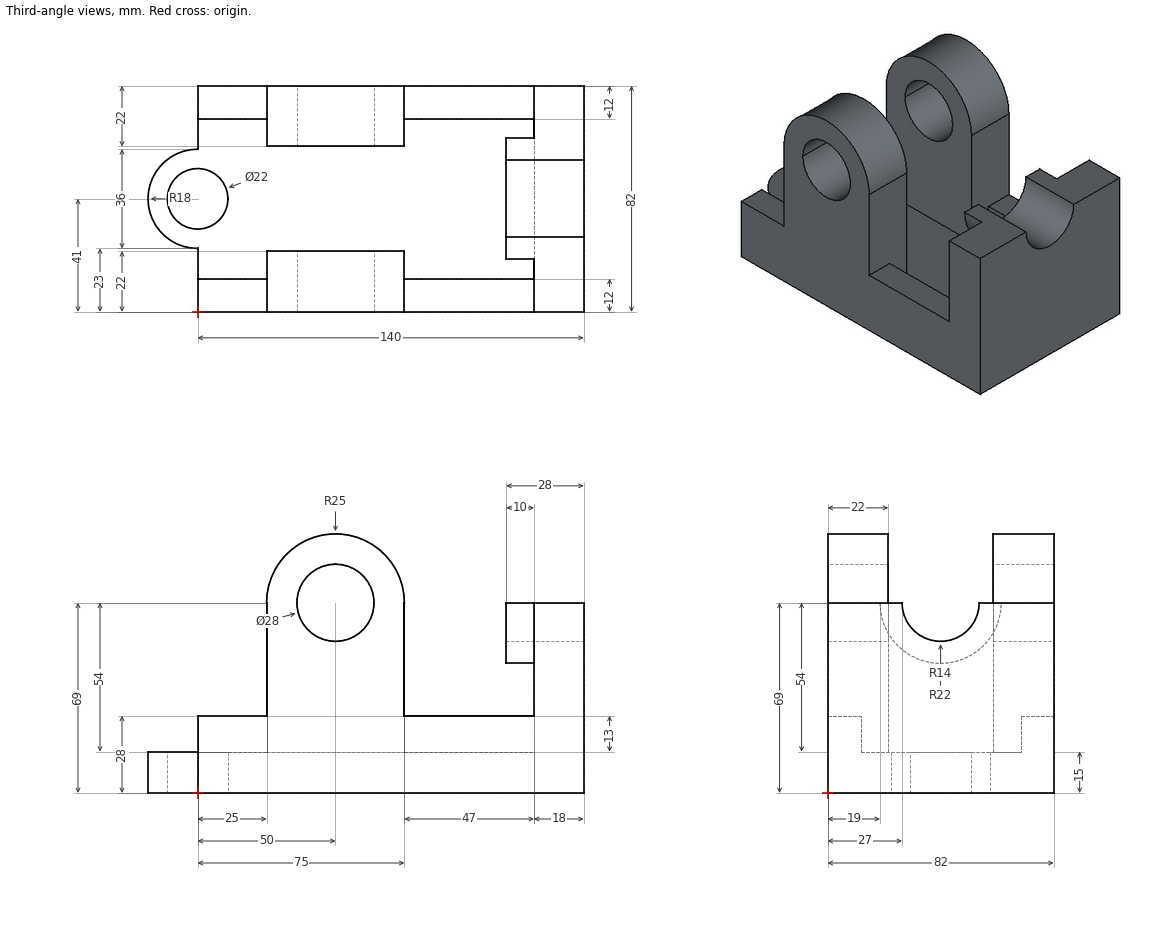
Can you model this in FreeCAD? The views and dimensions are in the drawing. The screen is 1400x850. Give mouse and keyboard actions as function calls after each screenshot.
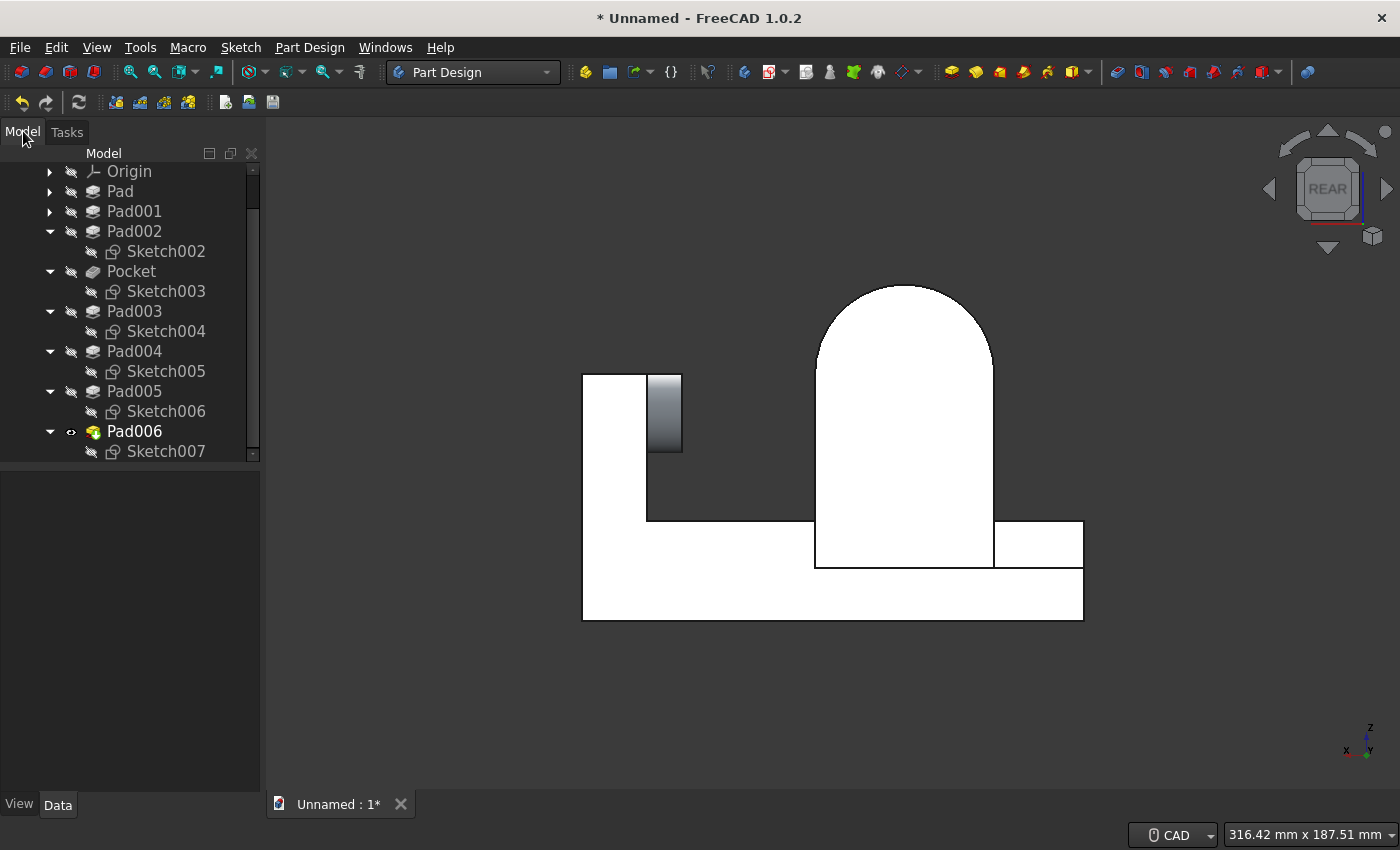
click(50, 172)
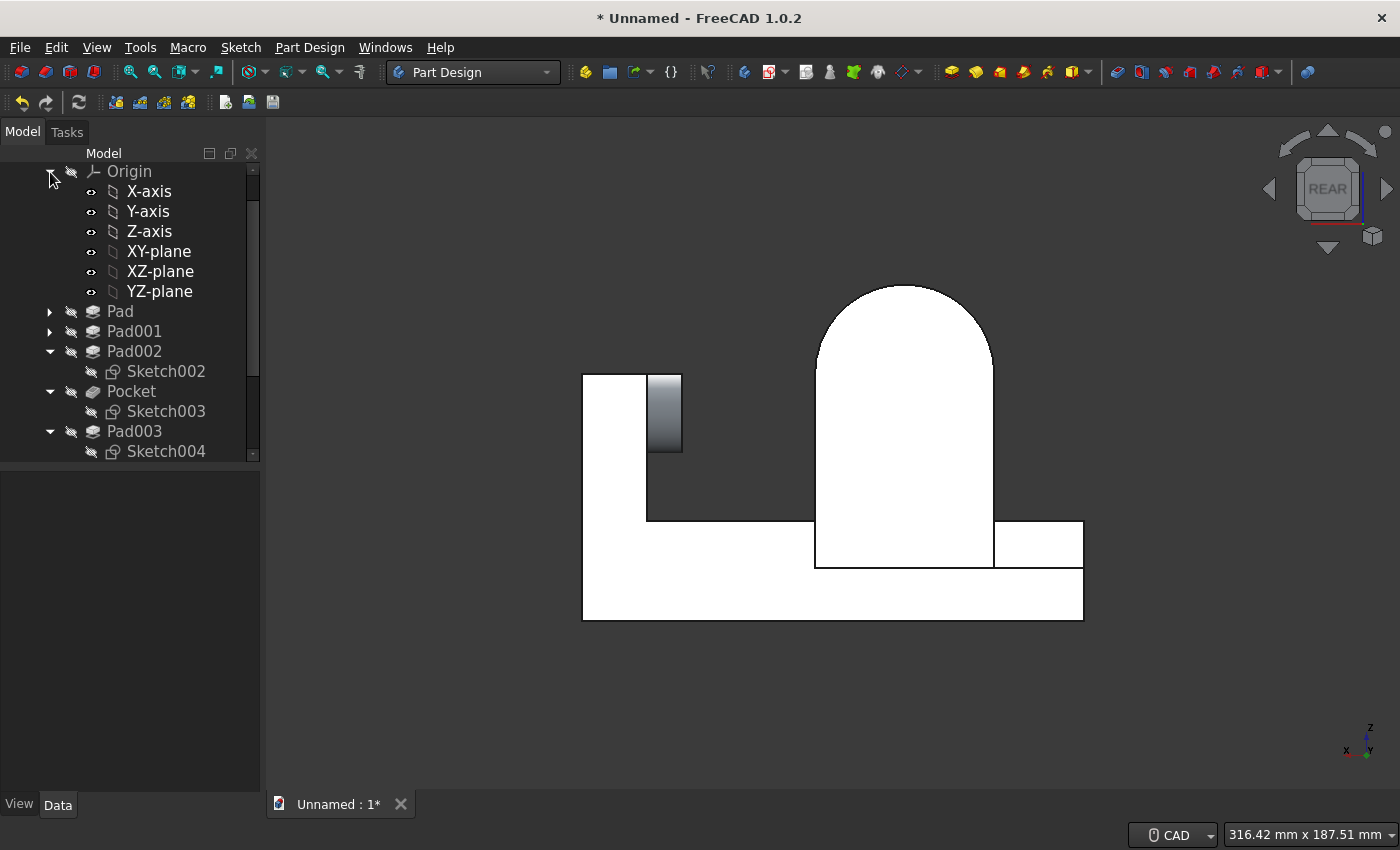
click(136, 272)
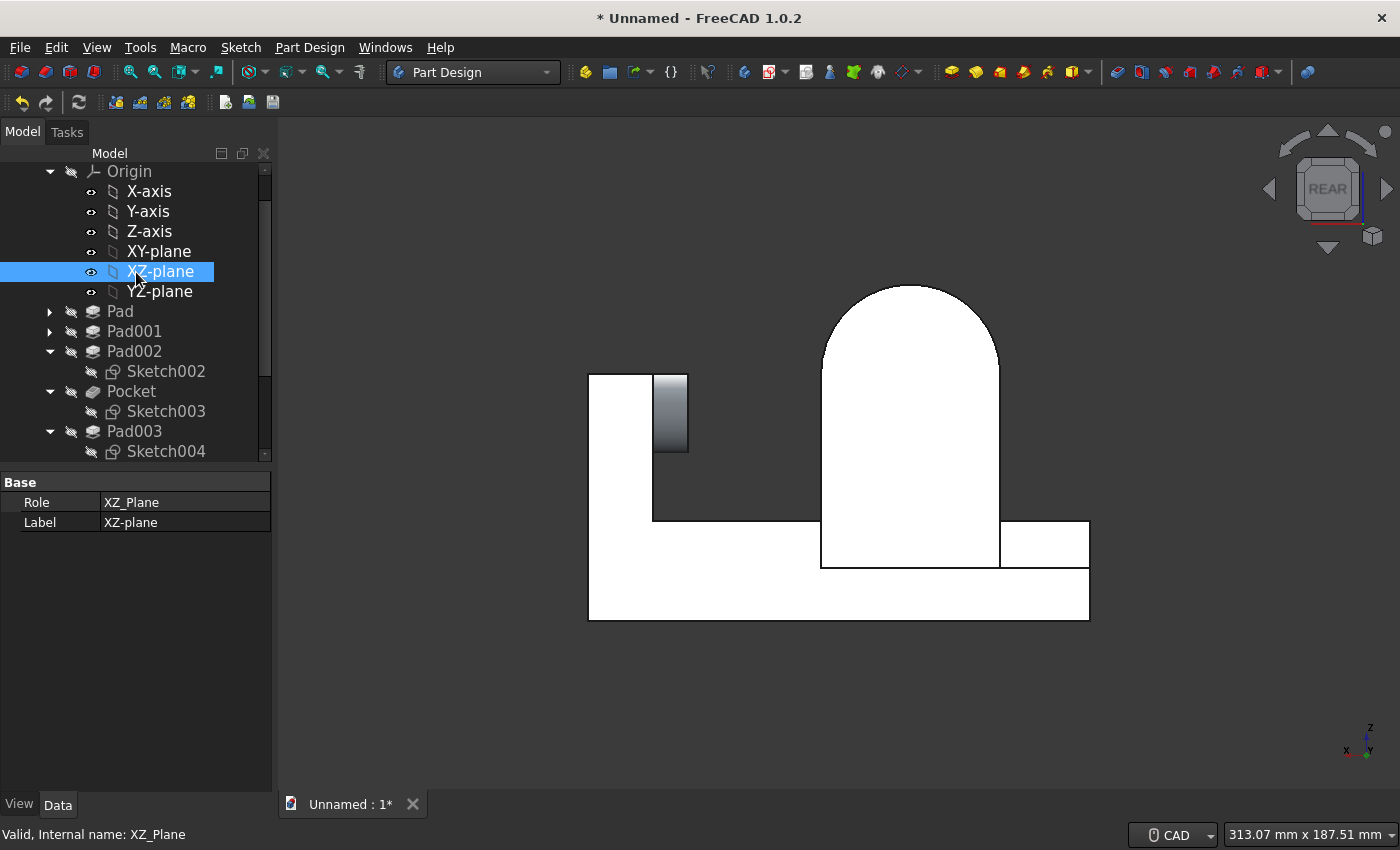
click(902, 72)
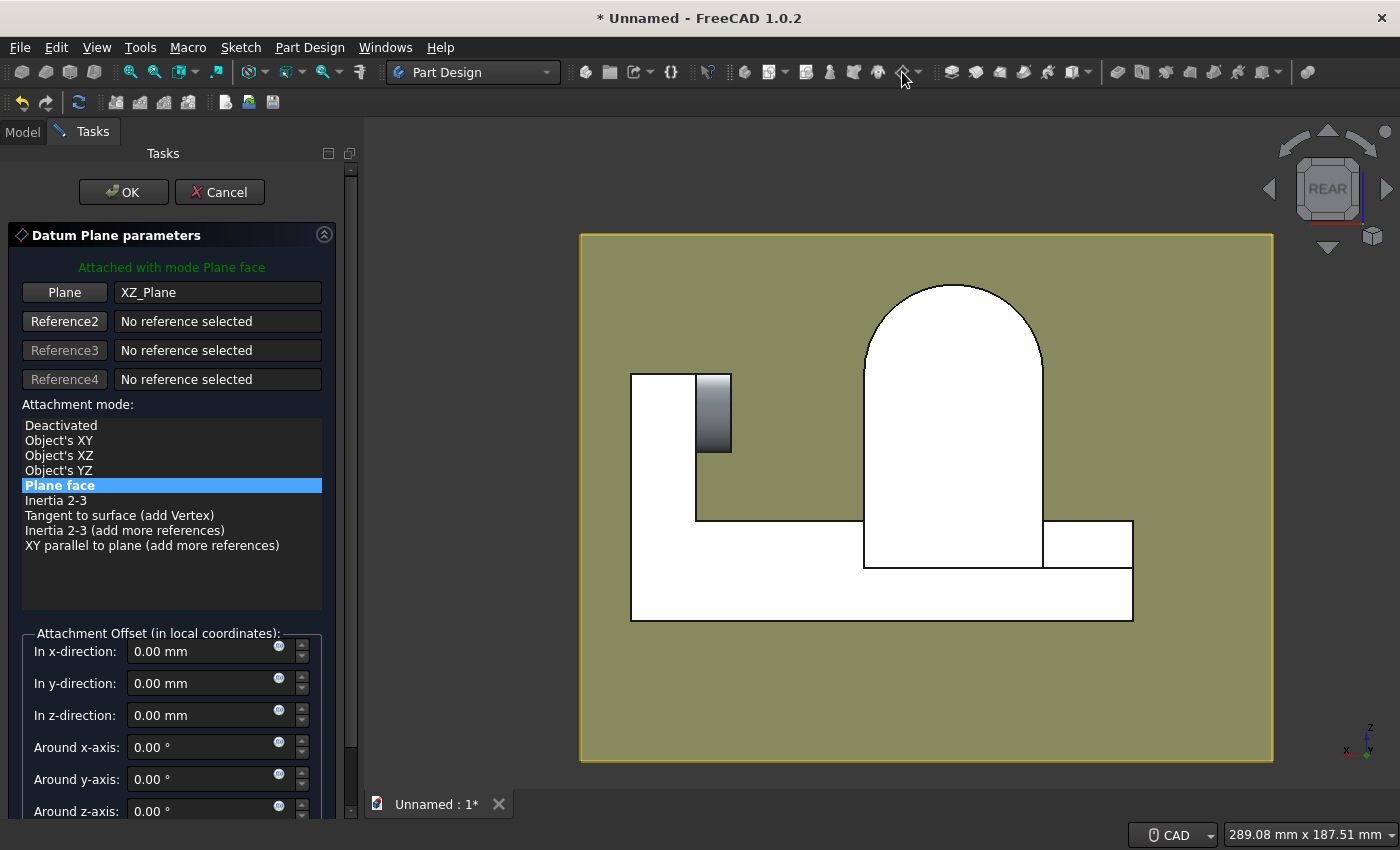
triple_click(210, 715)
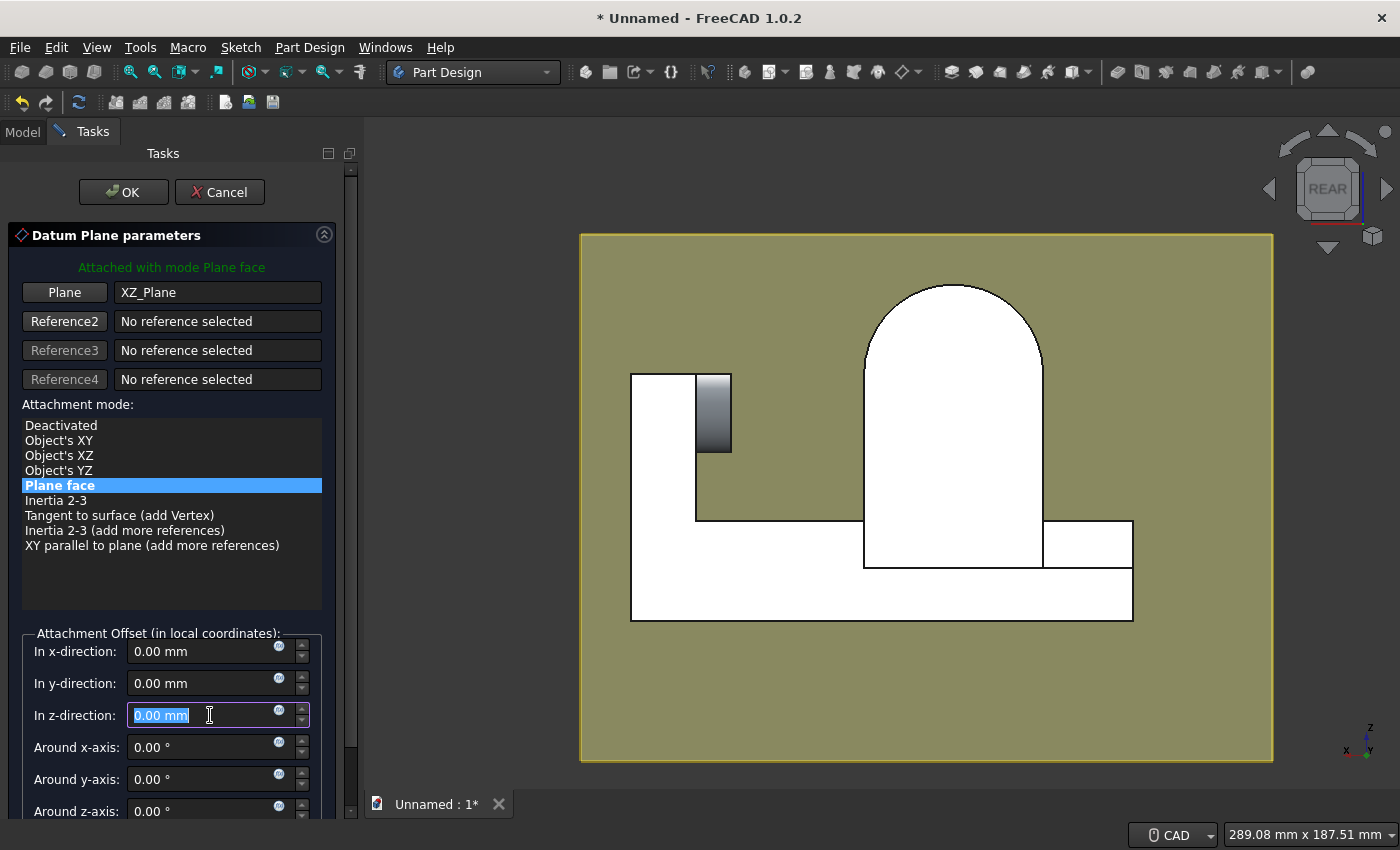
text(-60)
key(Tab)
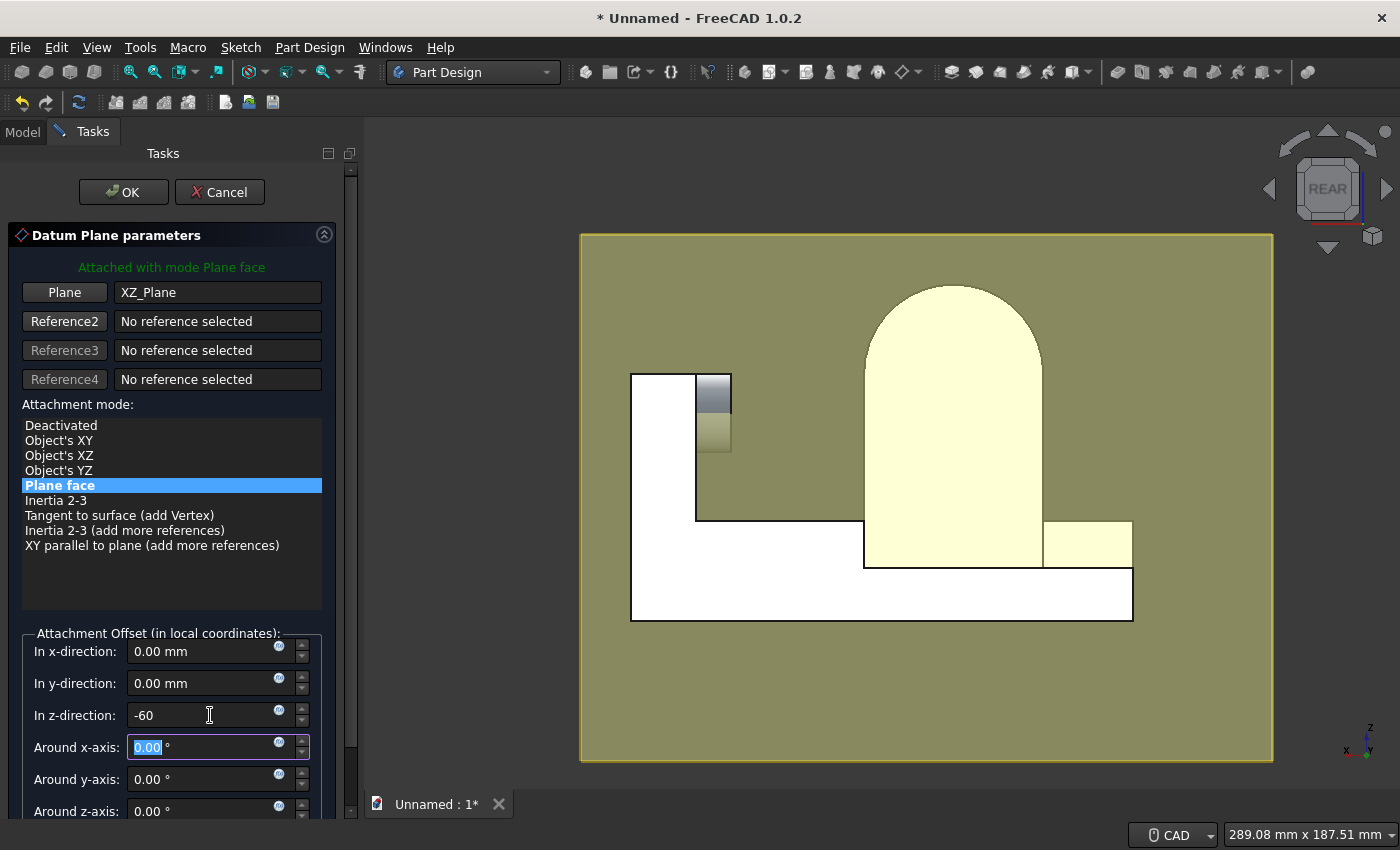
click(124, 192)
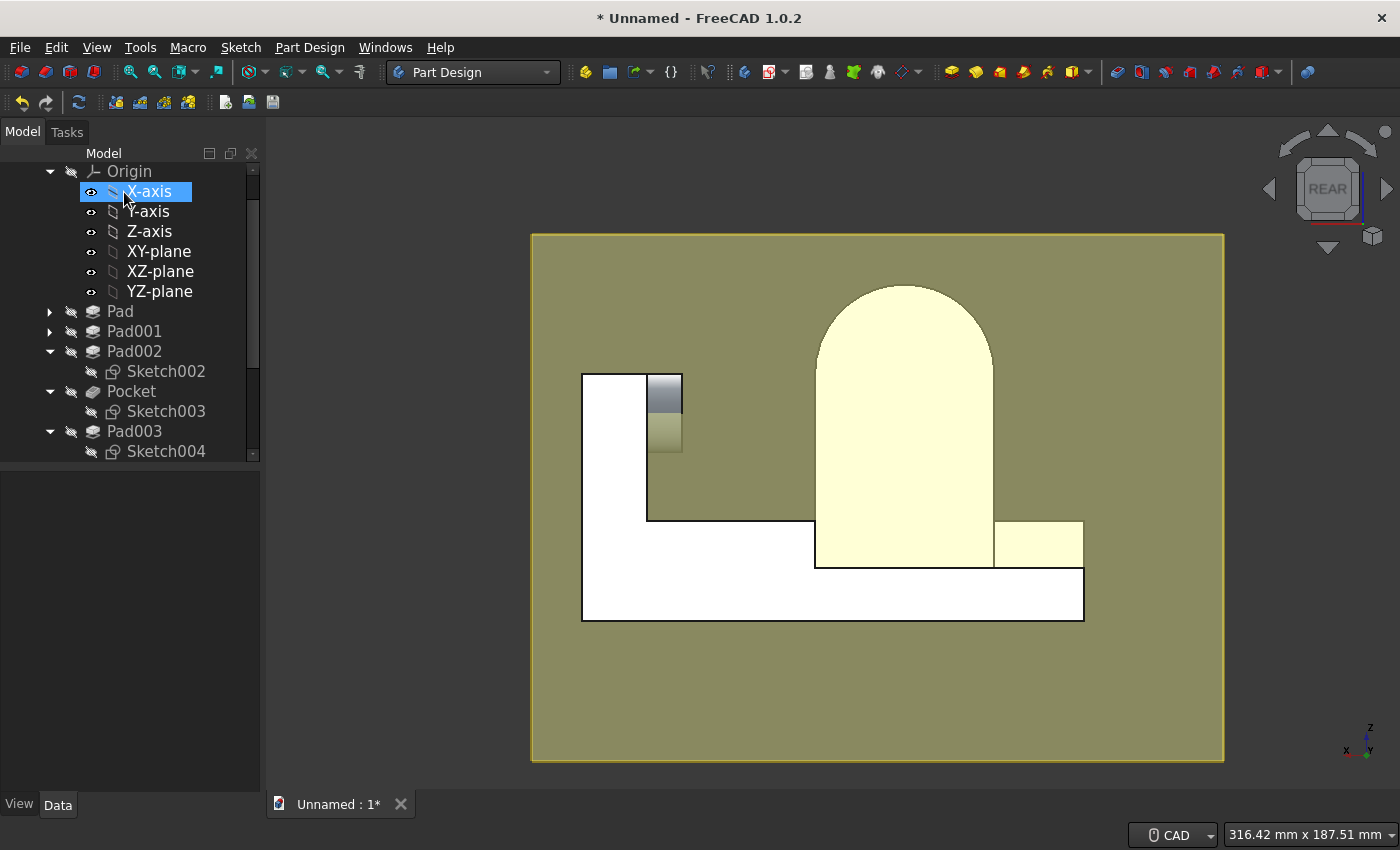
scroll(140, 307, down, 3)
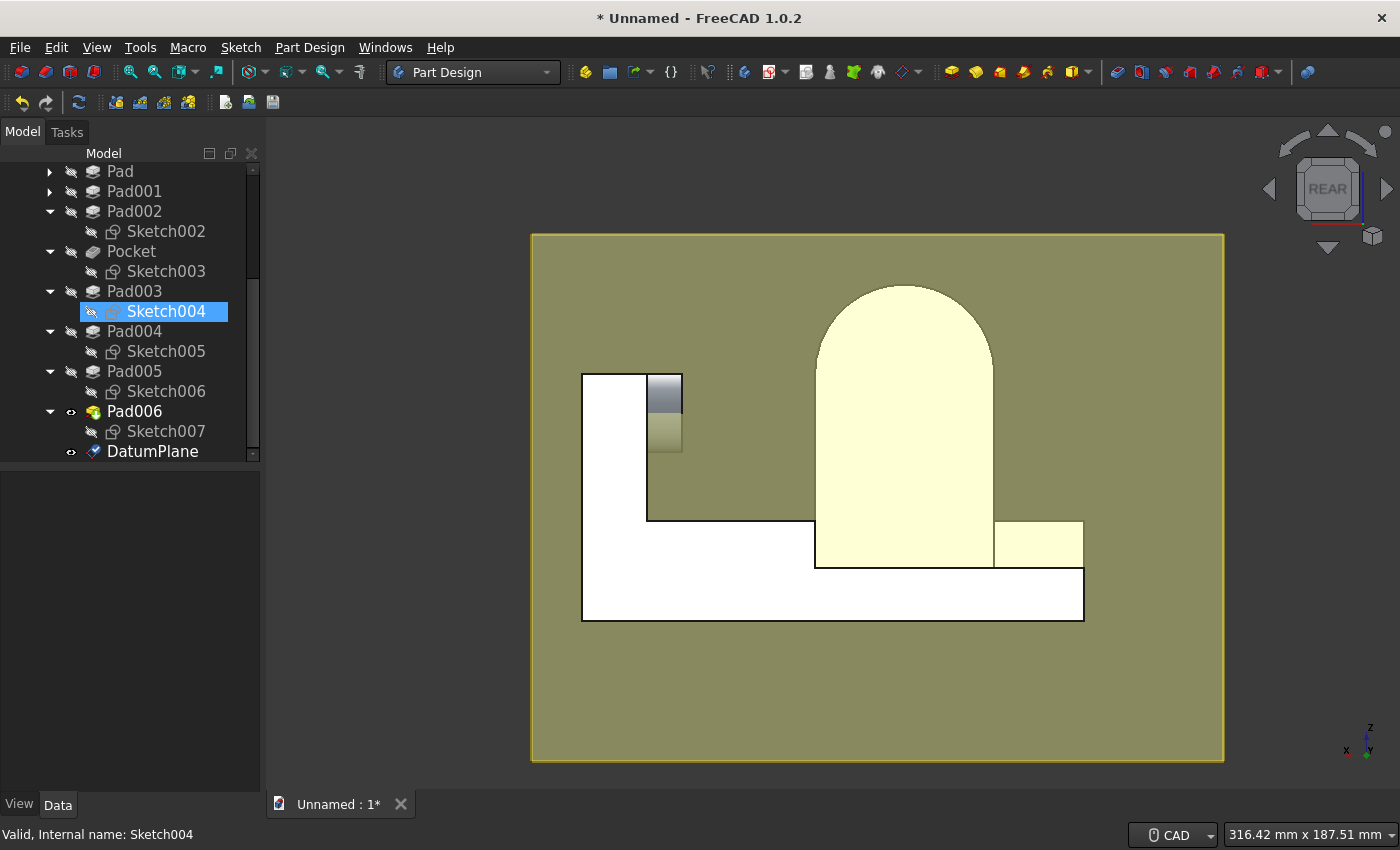
click(116, 452)